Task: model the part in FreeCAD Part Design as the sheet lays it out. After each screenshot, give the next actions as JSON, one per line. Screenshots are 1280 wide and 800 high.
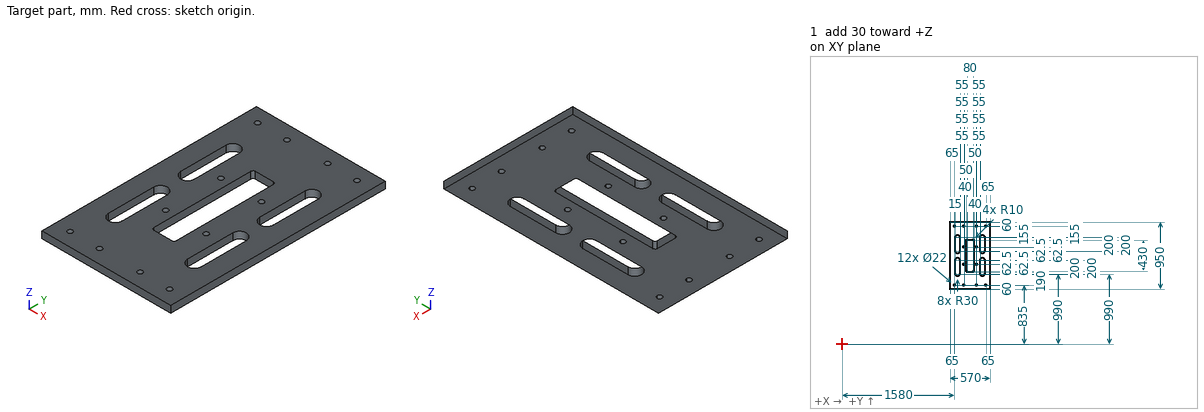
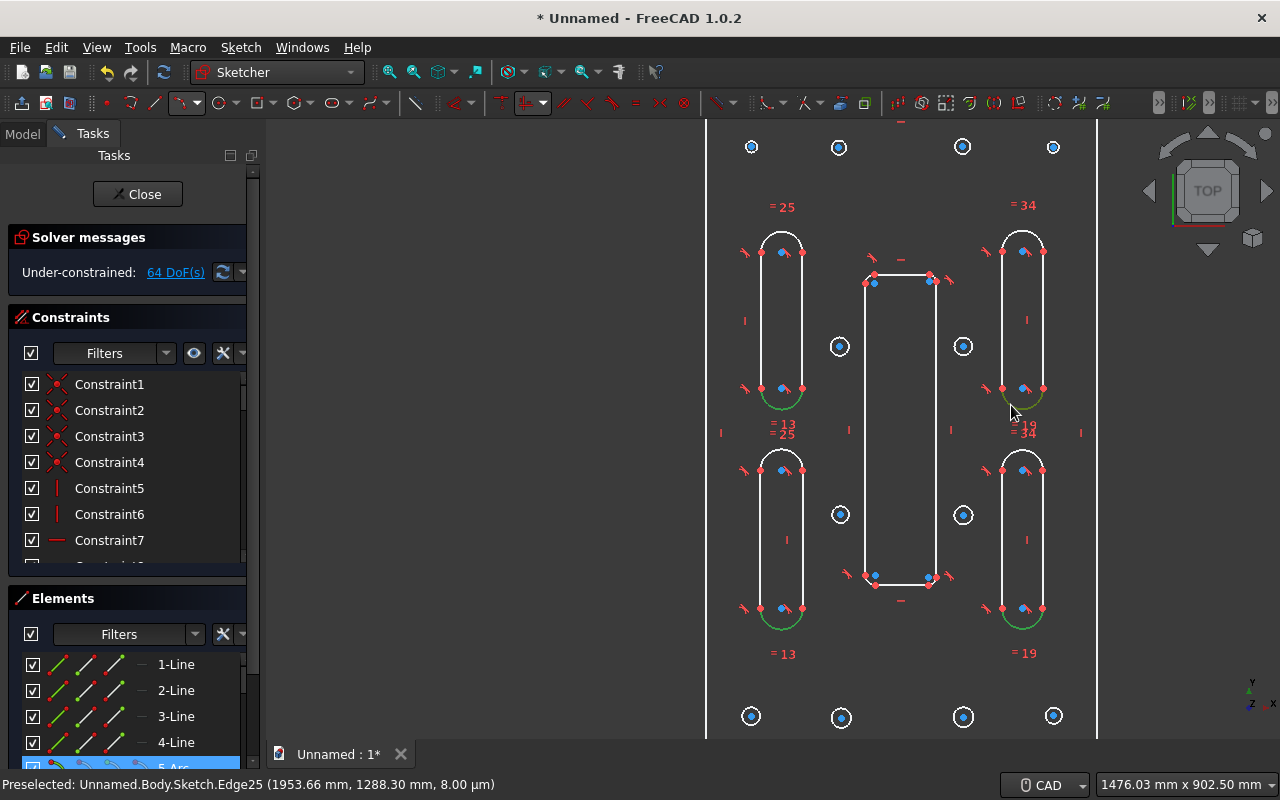
{"action": "left_click", "coordinate": [636, 104]}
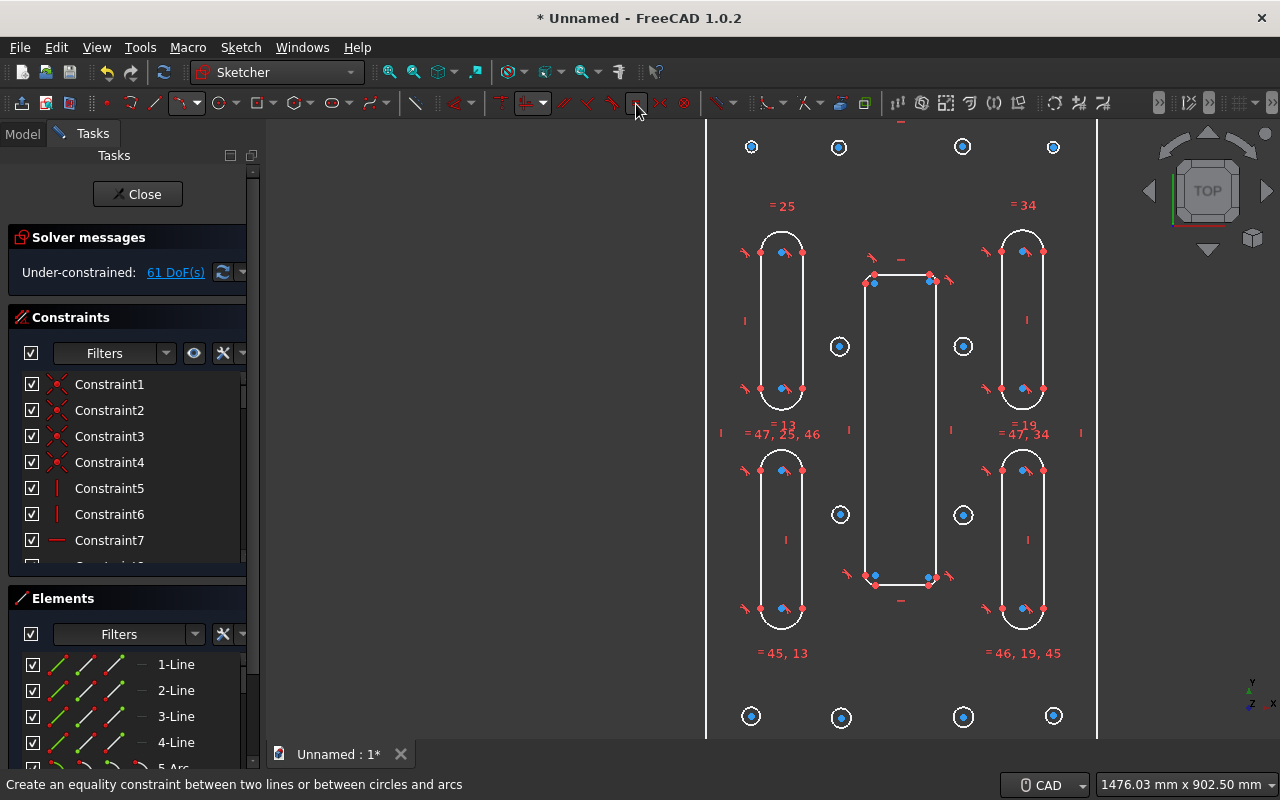
{"action": "scroll", "coordinate": [868, 582], "scroll_direction": "up", "scroll_amount": 3}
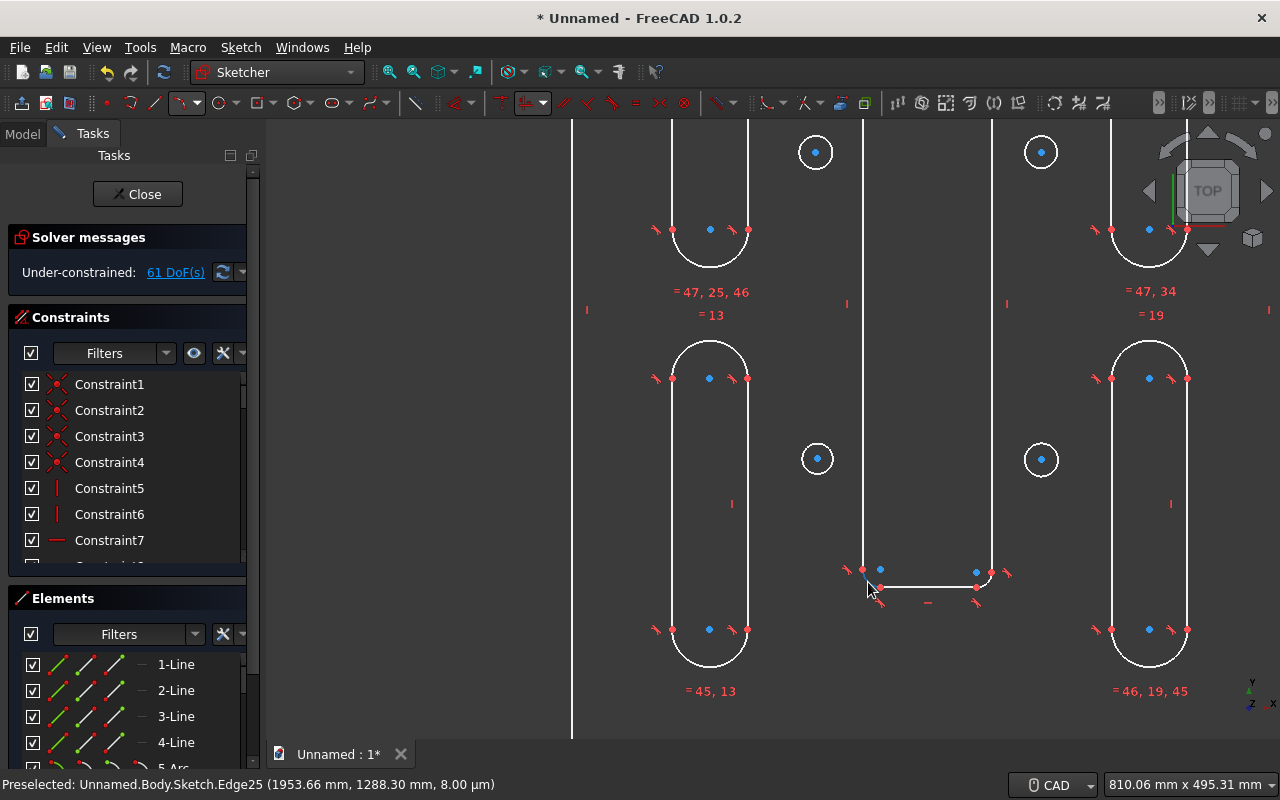
{"action": "left_click", "coordinate": [868, 582]}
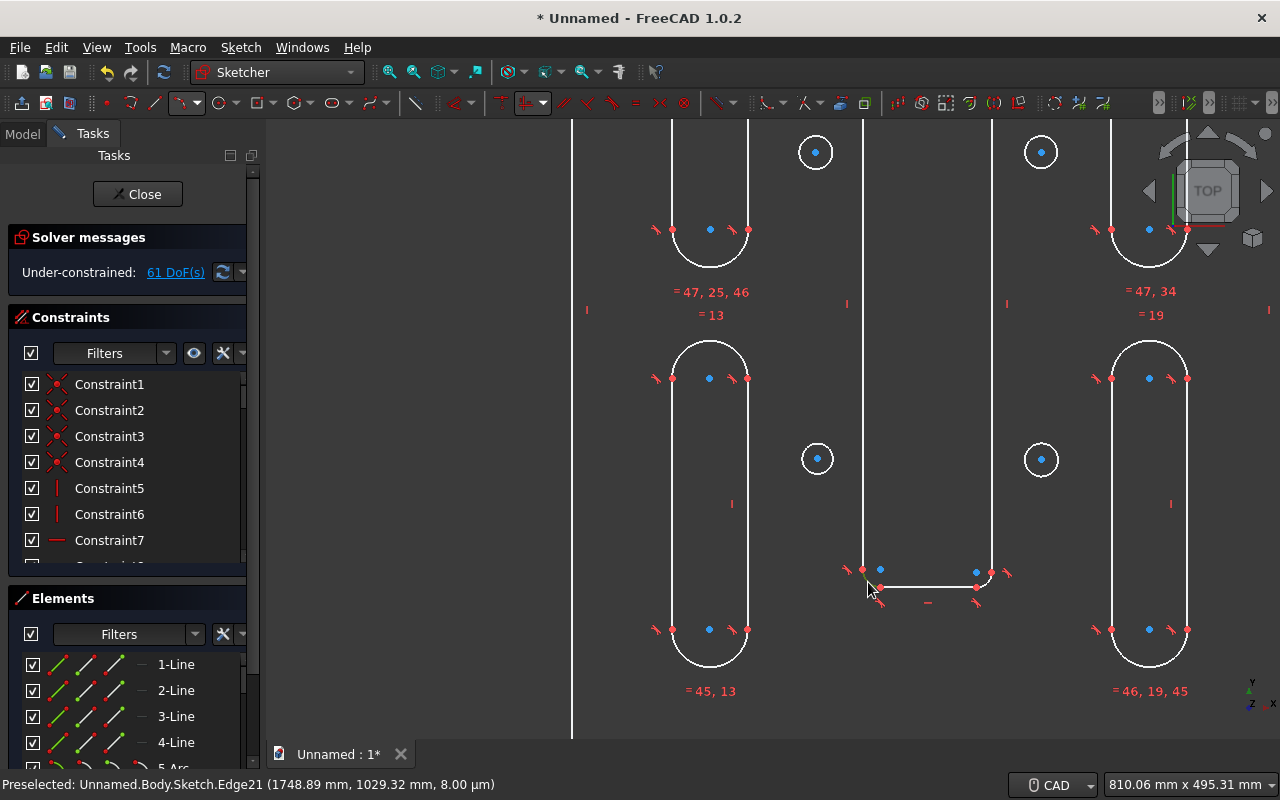
{"action": "scroll", "coordinate": [887, 338], "scroll_direction": "down", "scroll_amount": 8}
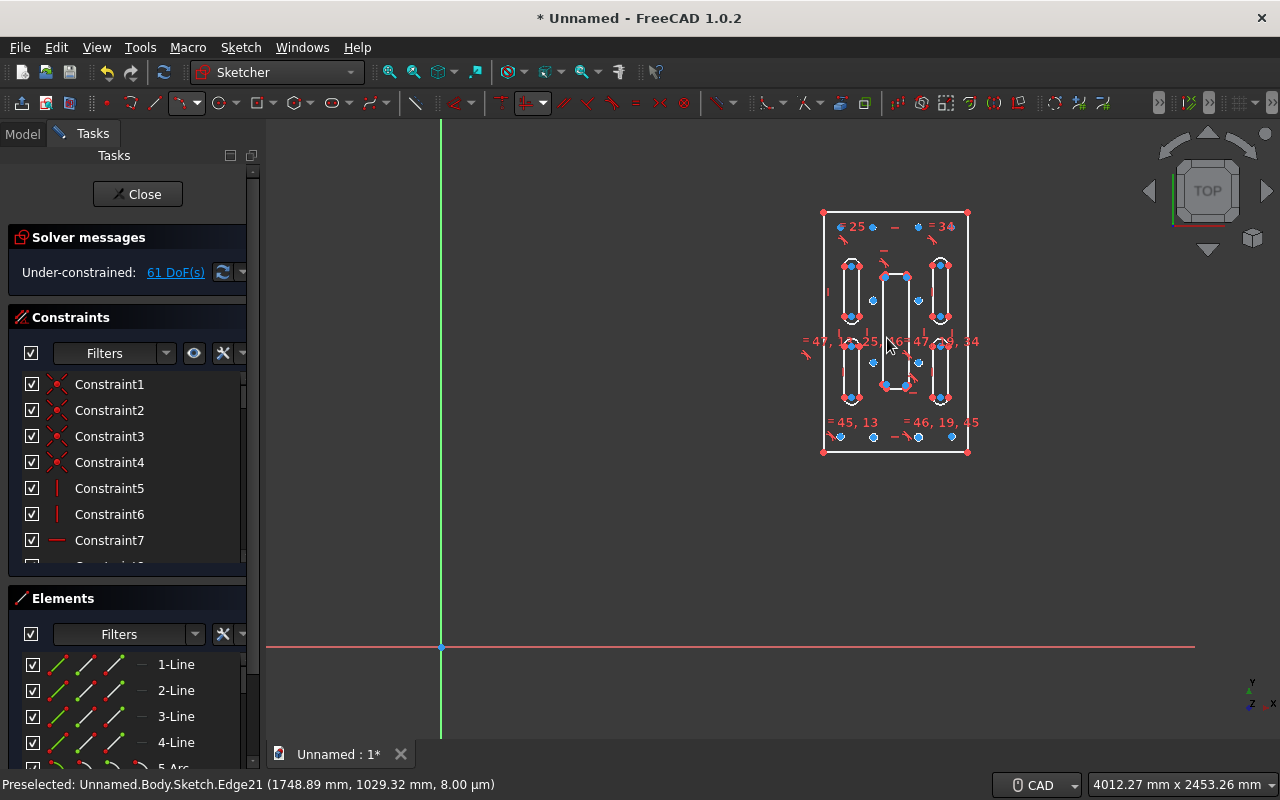
{"action": "scroll", "coordinate": [884, 275], "scroll_direction": "up", "scroll_amount": 9}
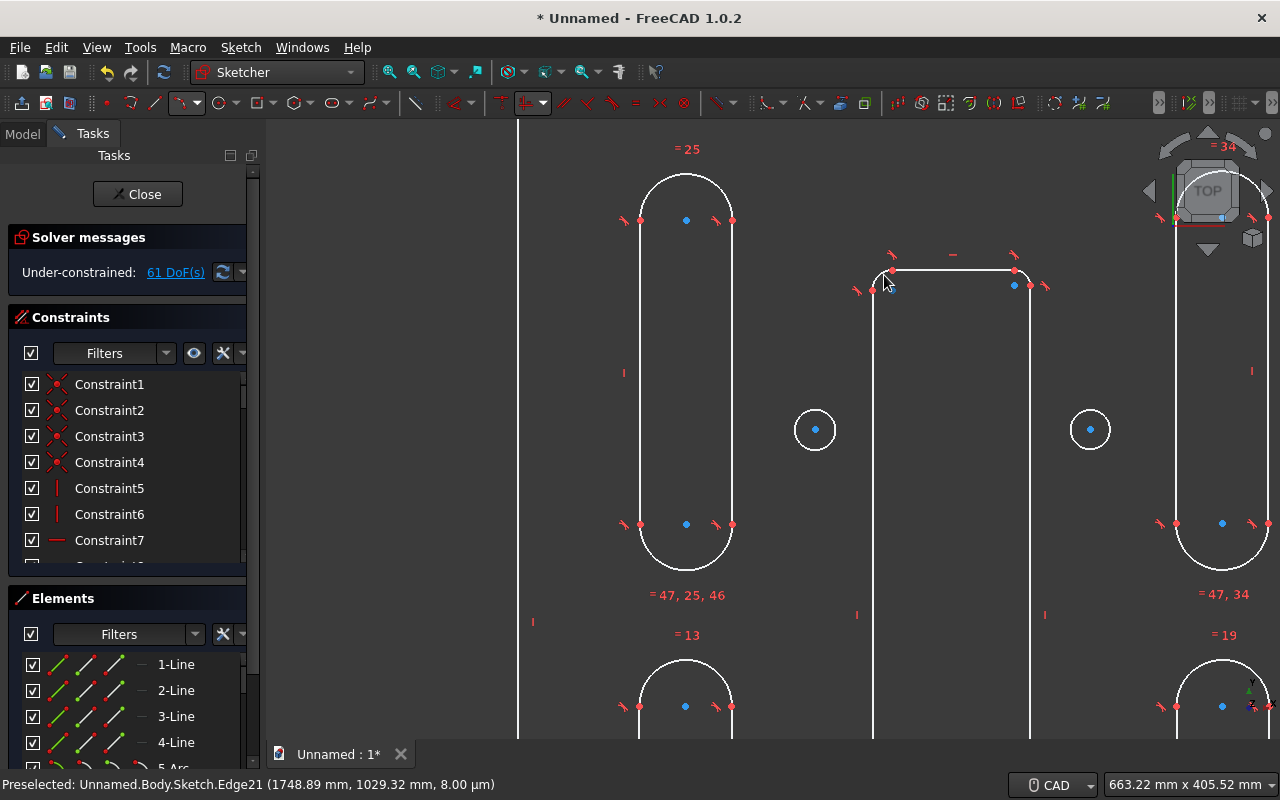
{"action": "left_click", "coordinate": [878, 276]}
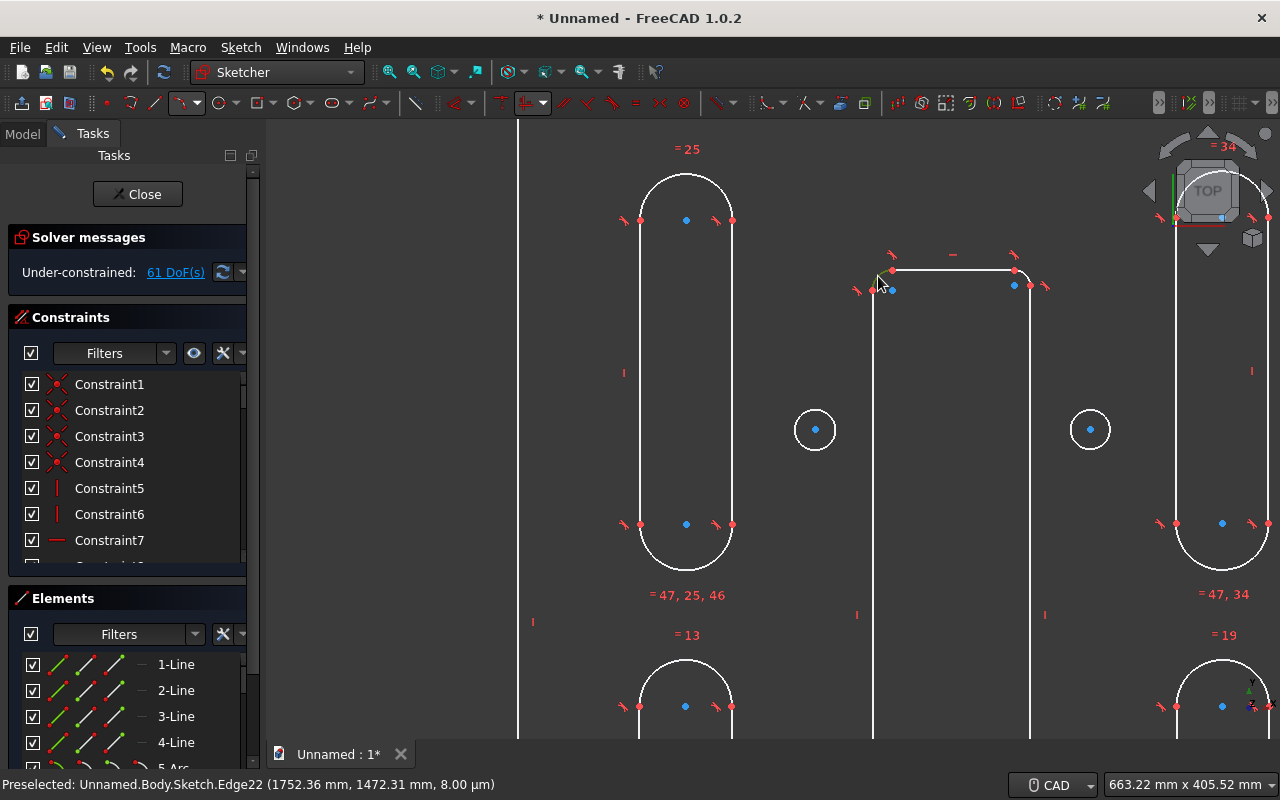
{"action": "left_click", "coordinate": [1025, 275]}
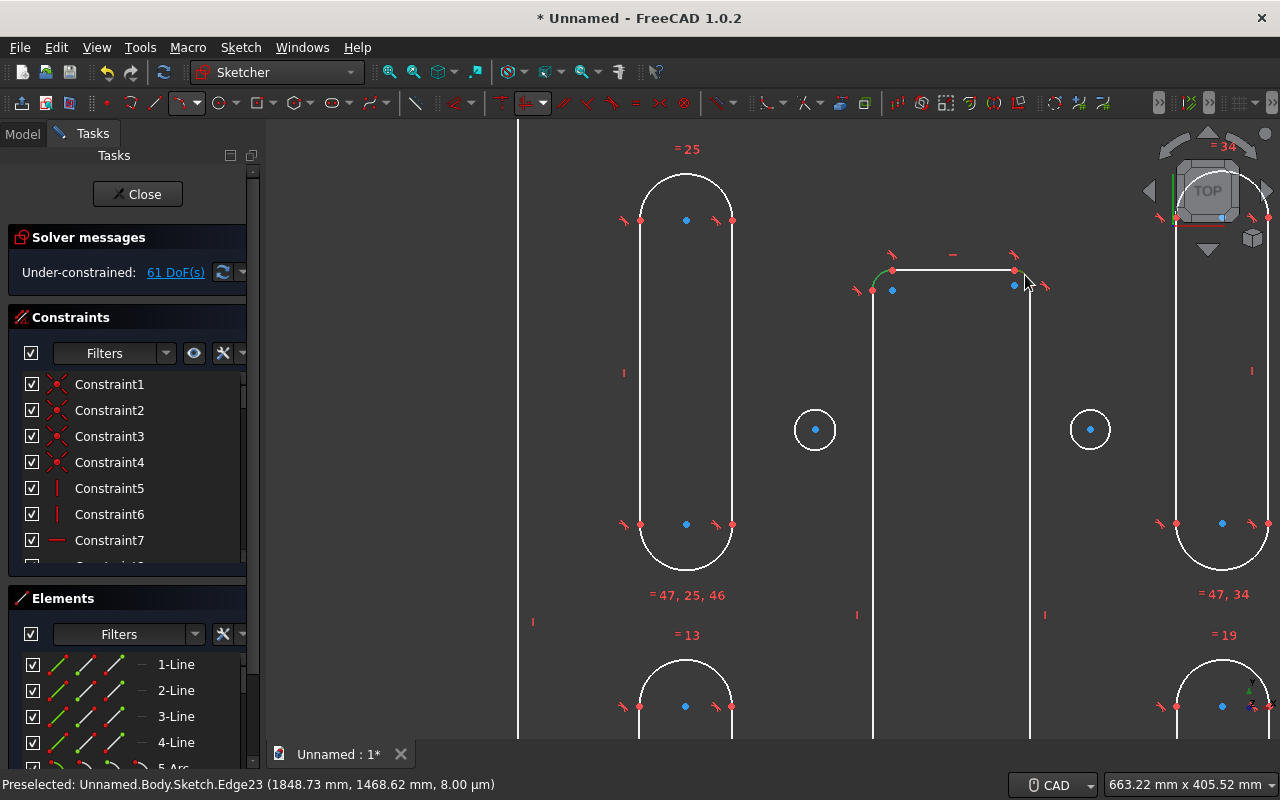
{"action": "scroll", "coordinate": [884, 275], "scroll_direction": "down", "scroll_amount": 9}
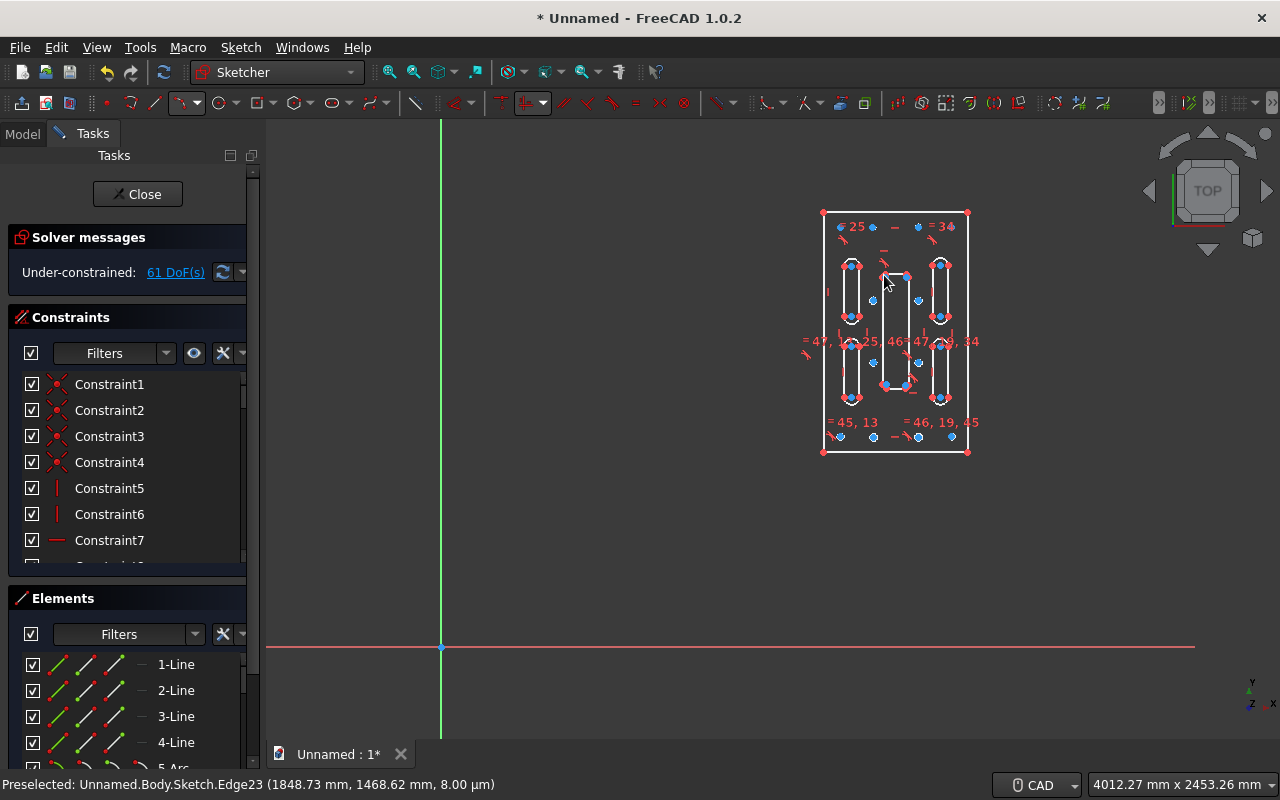
{"action": "scroll", "coordinate": [908, 388], "scroll_direction": "up", "scroll_amount": 9}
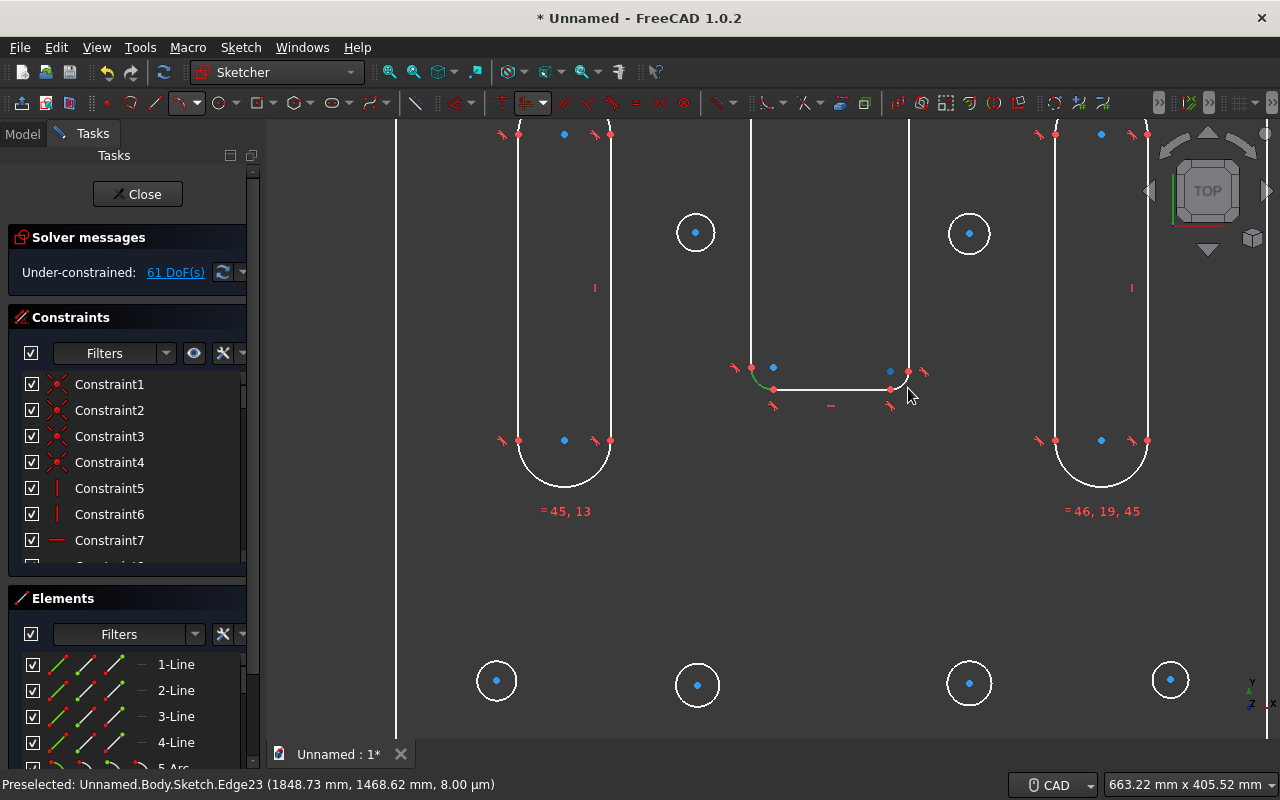
{"action": "left_click", "coordinate": [903, 384]}